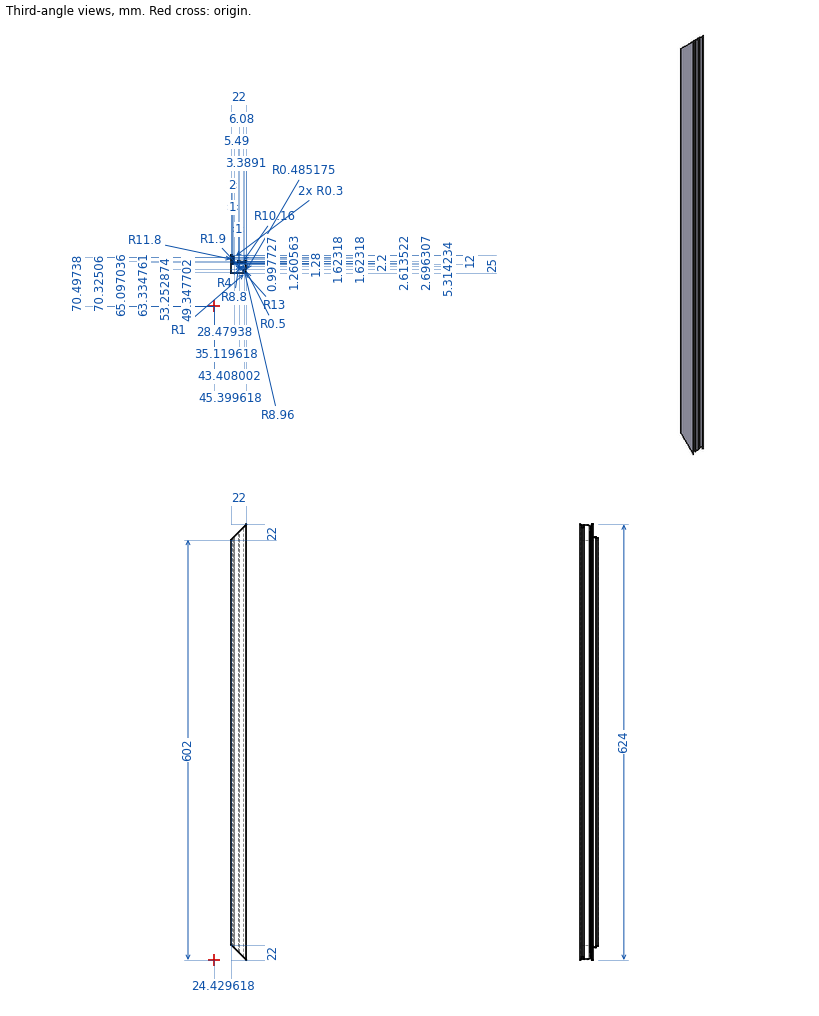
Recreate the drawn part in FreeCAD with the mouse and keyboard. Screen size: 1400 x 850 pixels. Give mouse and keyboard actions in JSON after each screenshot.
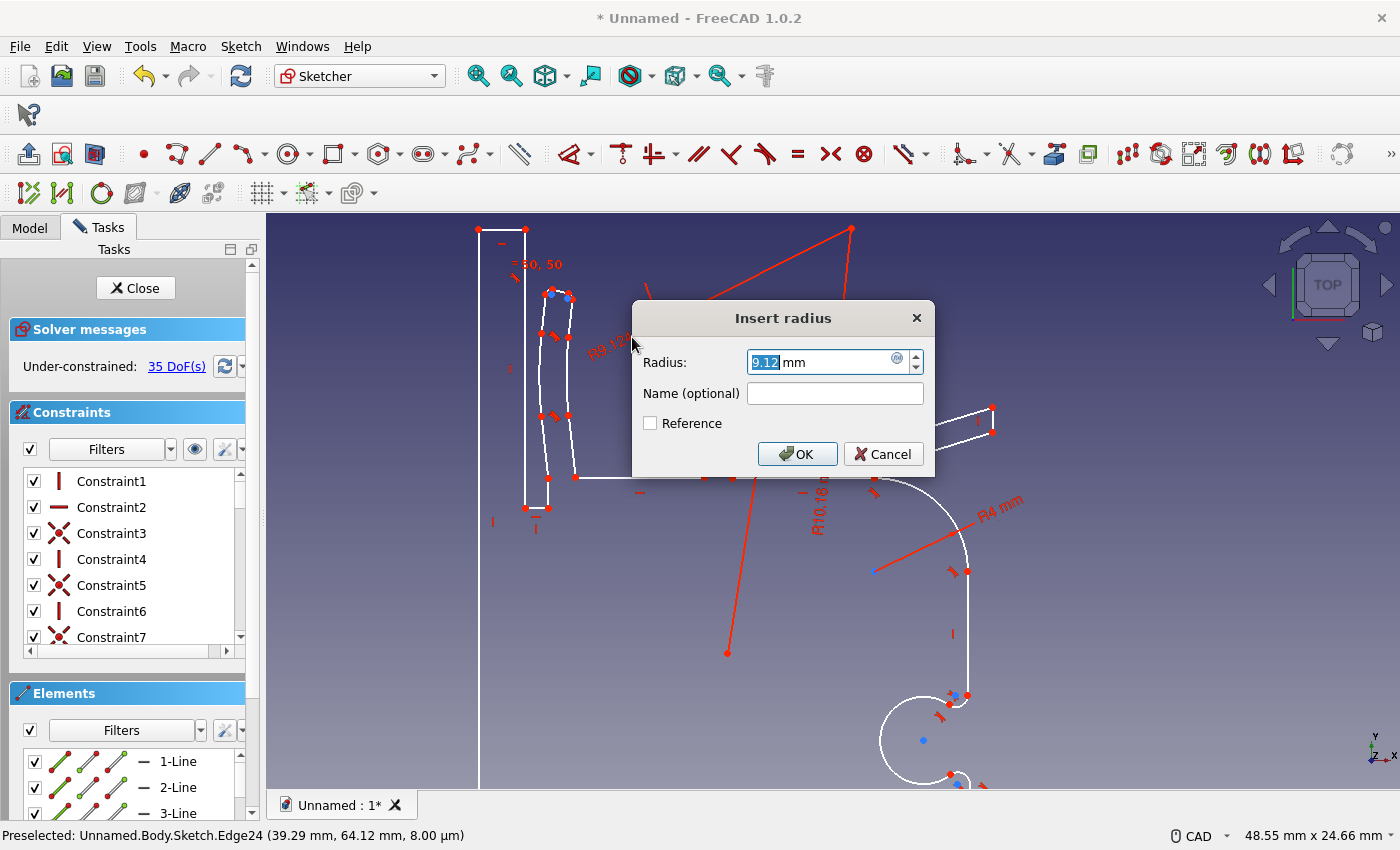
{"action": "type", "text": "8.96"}
{"action": "key", "text": "Return"}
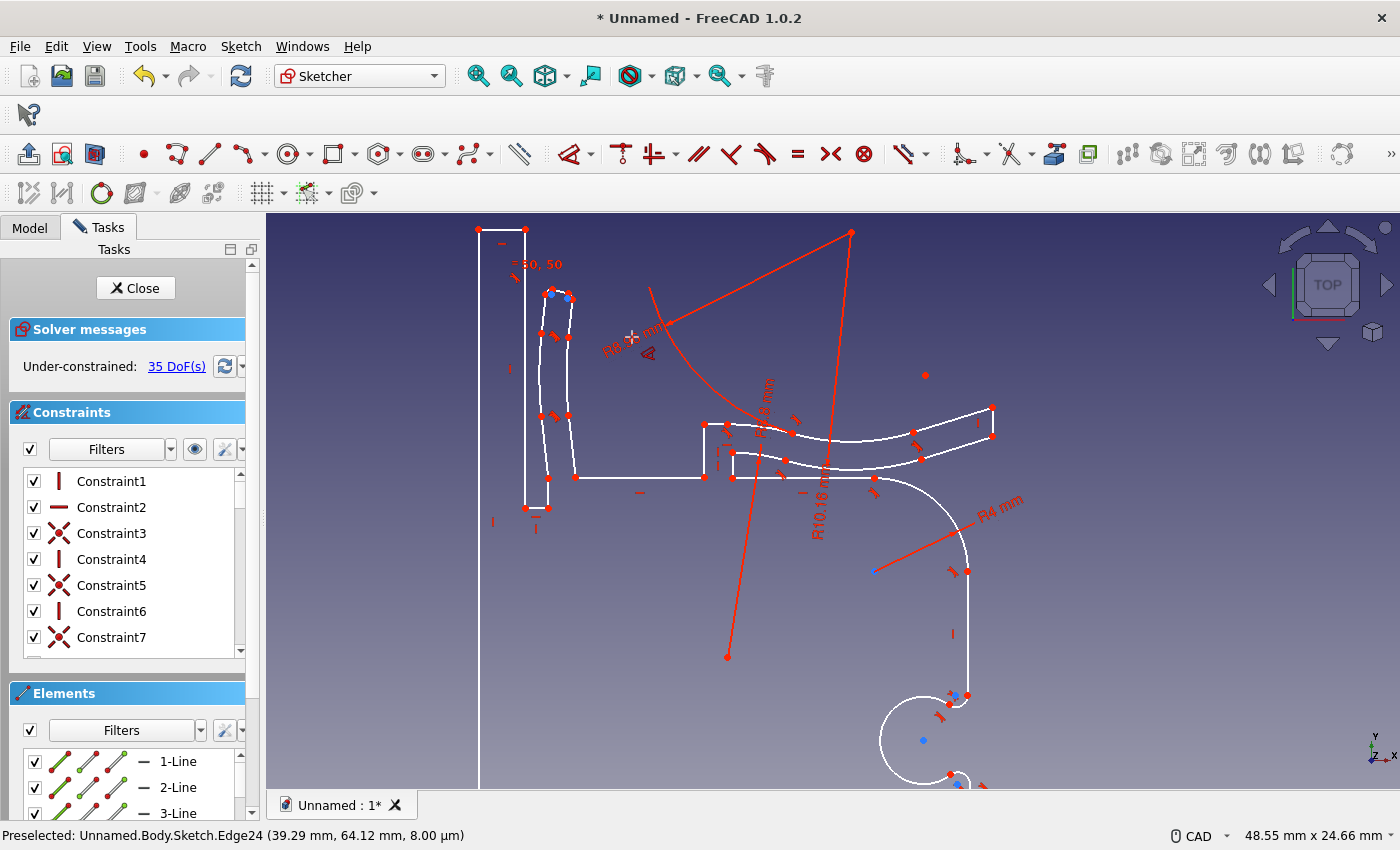
{"action": "left_click", "coordinate": [567, 361]}
{"action": "left_click", "coordinate": [575, 549]}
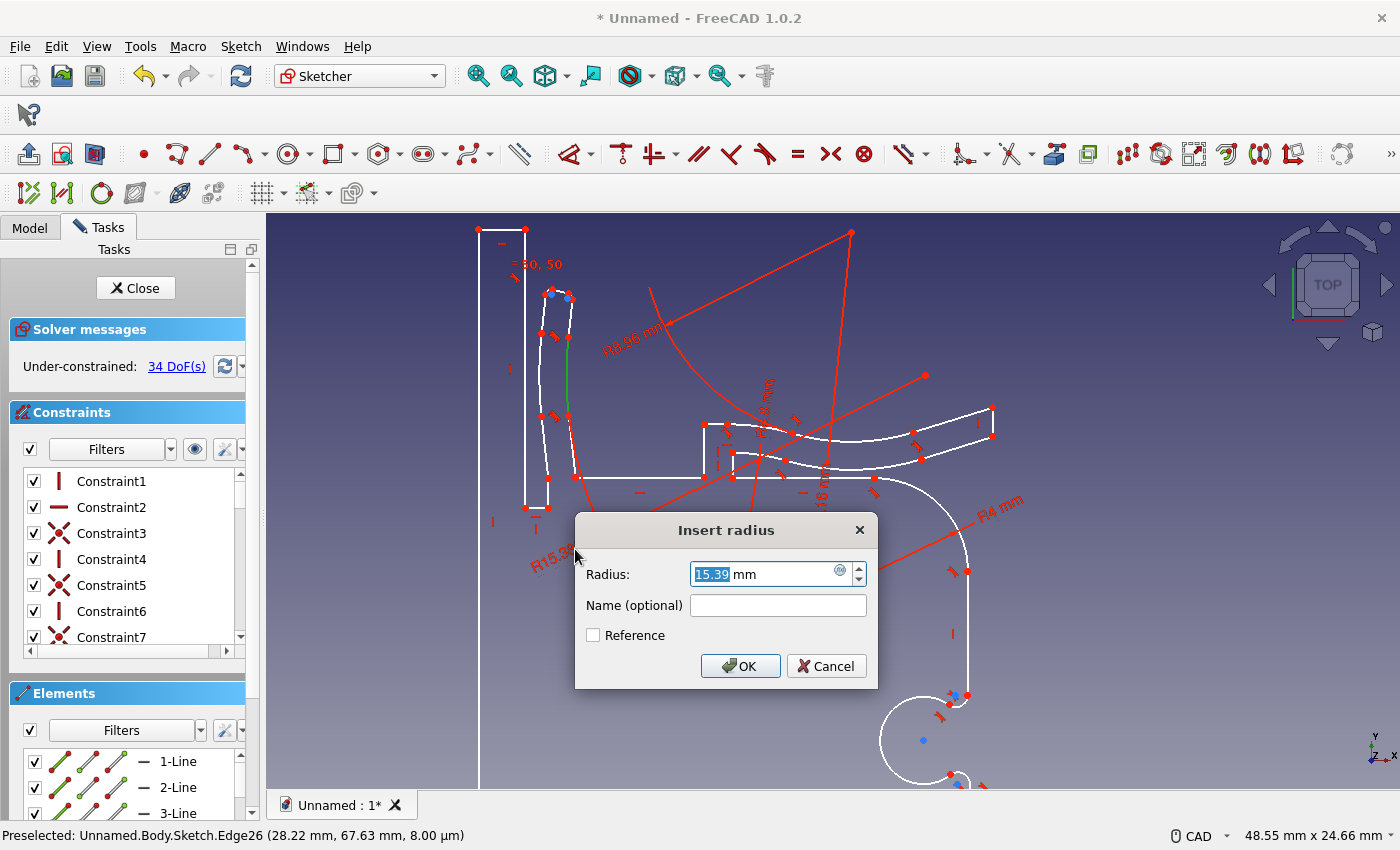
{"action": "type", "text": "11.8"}
{"action": "key", "text": "Return"}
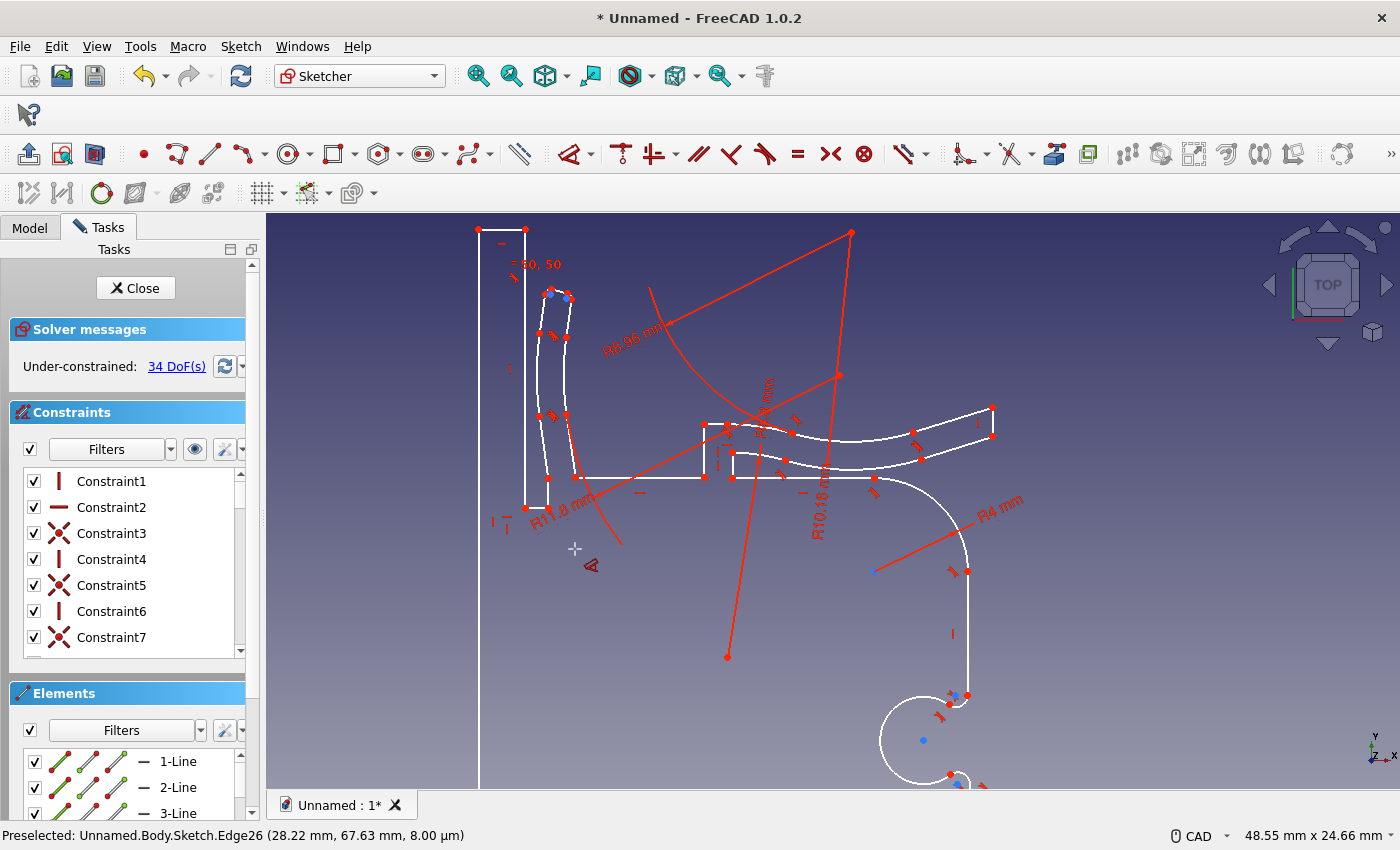
{"action": "scroll", "coordinate": [571, 296], "scroll_direction": "up", "scroll_amount": 9}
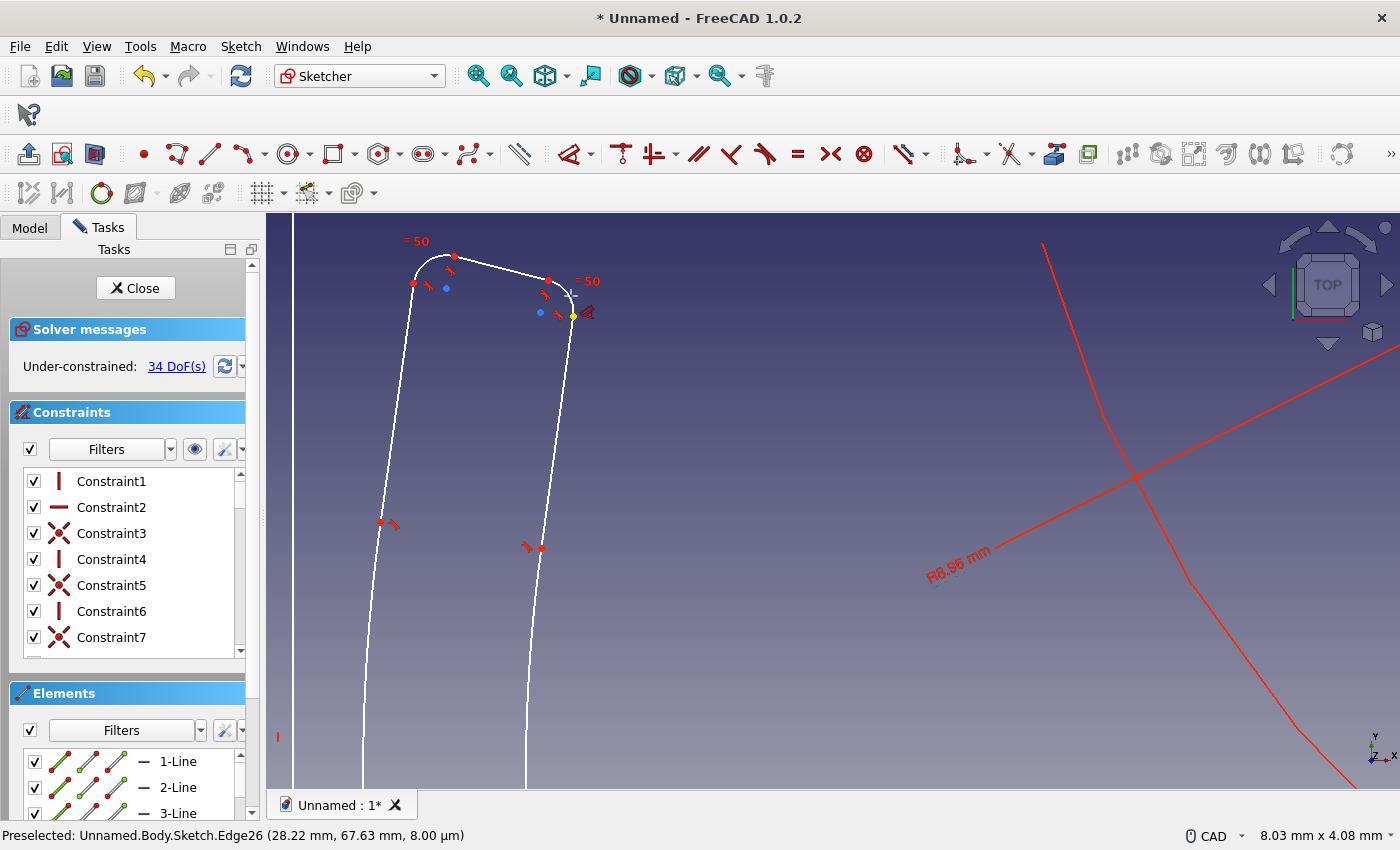
{"action": "left_click", "coordinate": [568, 294]}
{"action": "left_click", "coordinate": [595, 276]}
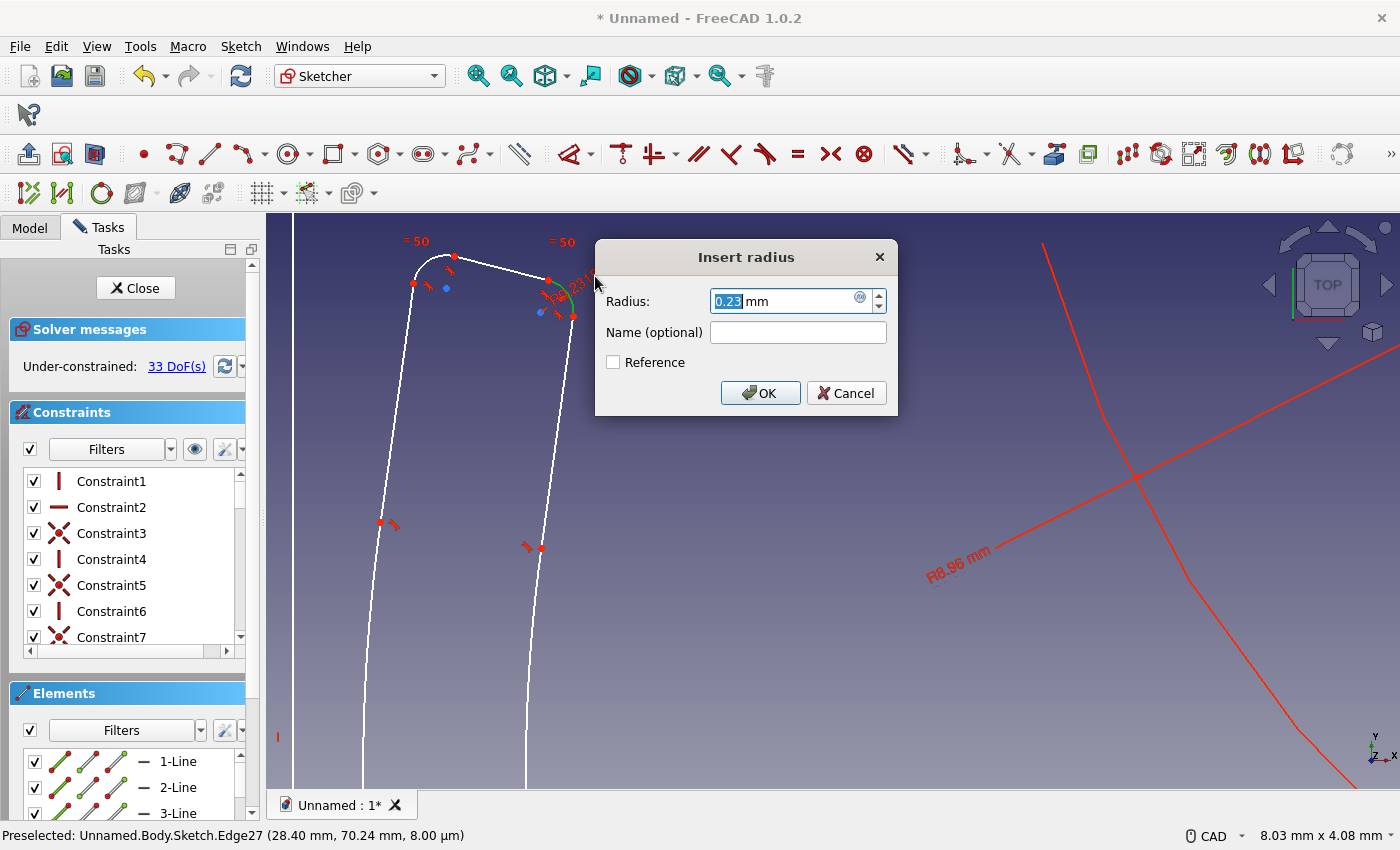
{"action": "type", "text": "0.3"}
{"action": "key", "text": "Return"}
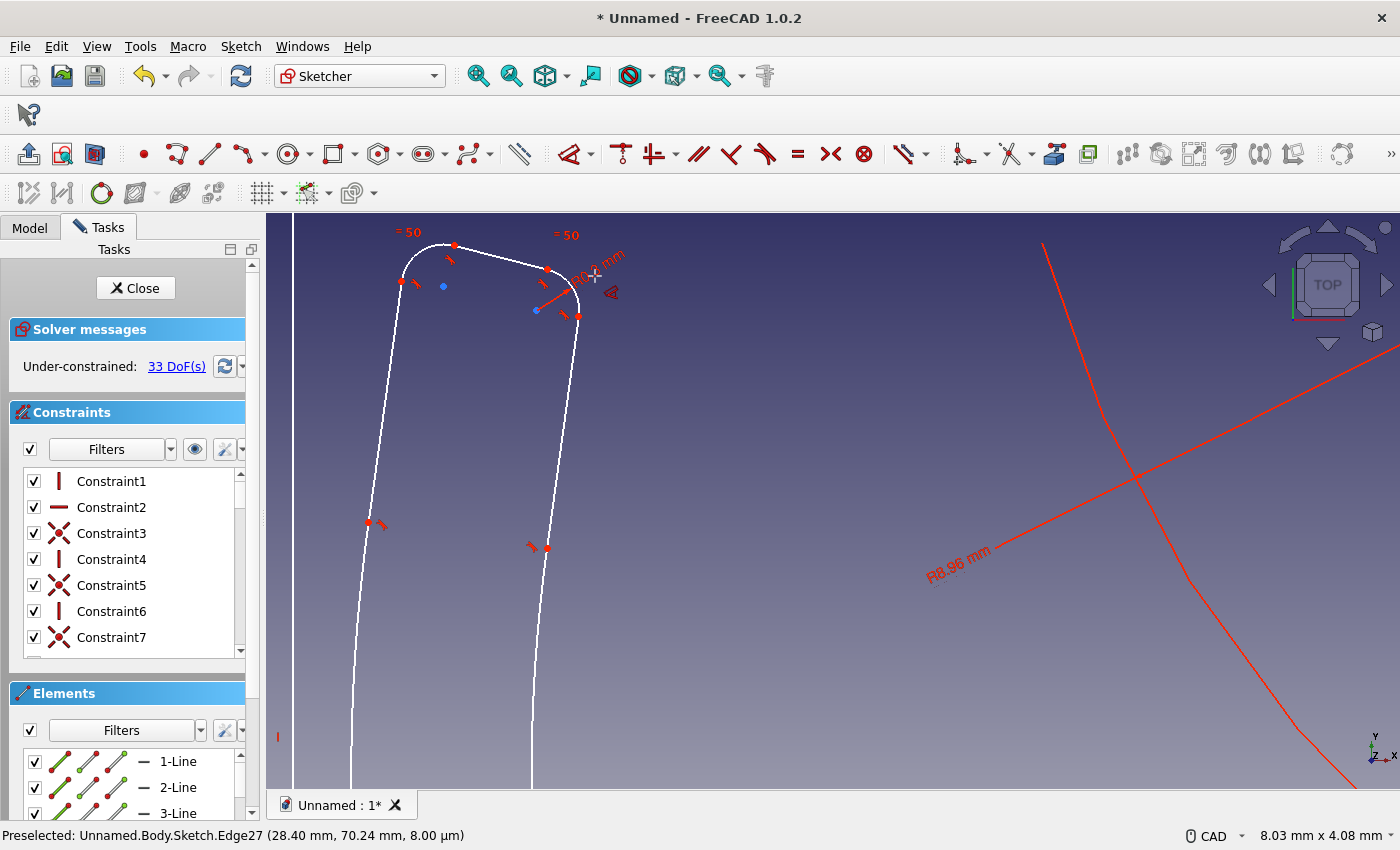
{"action": "scroll", "coordinate": [665, 358], "scroll_direction": "down", "scroll_amount": 11}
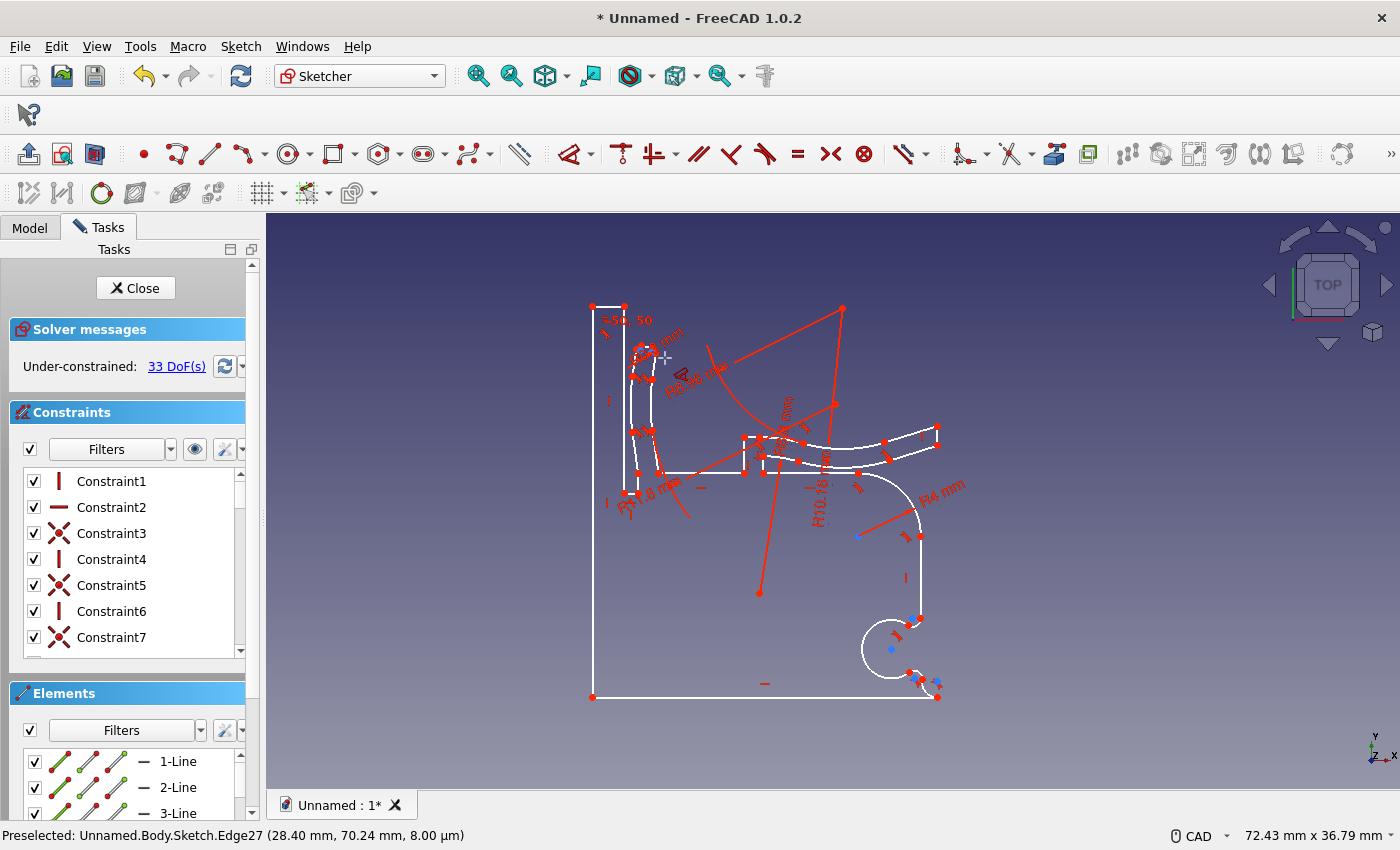
{"action": "scroll", "coordinate": [631, 393], "scroll_direction": "up", "scroll_amount": 4}